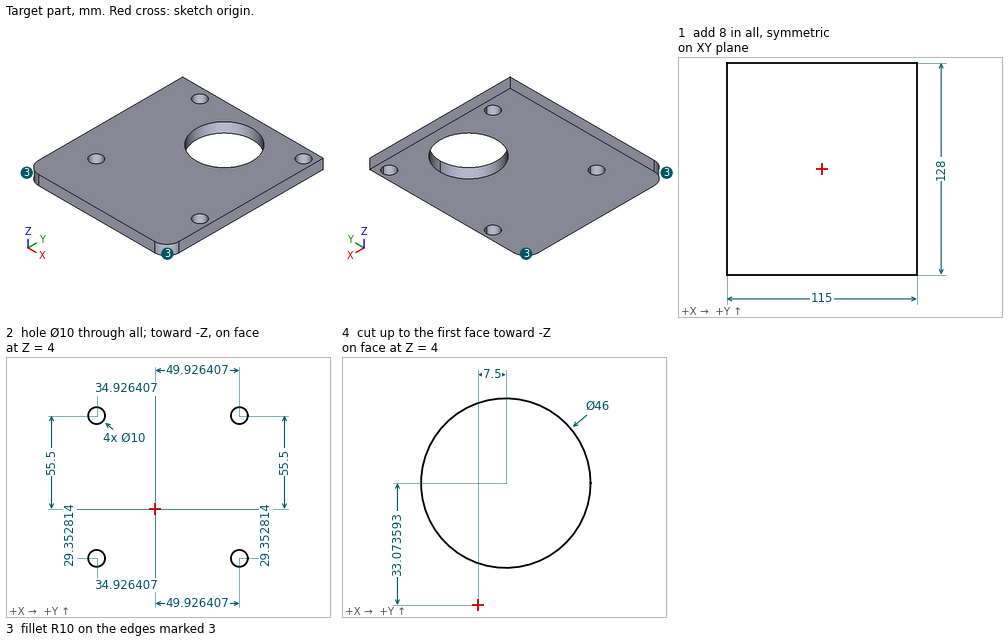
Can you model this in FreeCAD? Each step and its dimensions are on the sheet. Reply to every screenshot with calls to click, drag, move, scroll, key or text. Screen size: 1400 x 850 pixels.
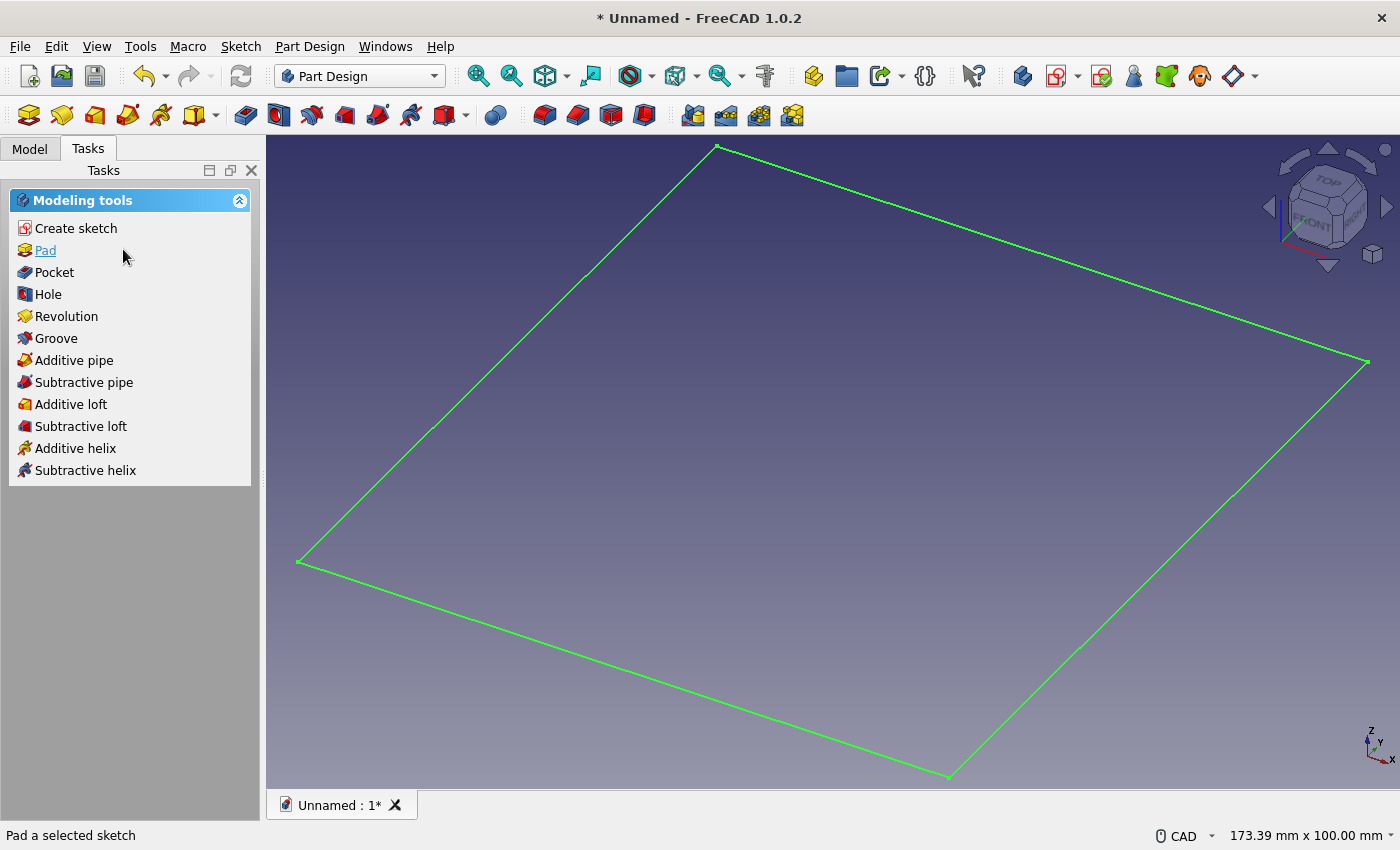
click(29, 116)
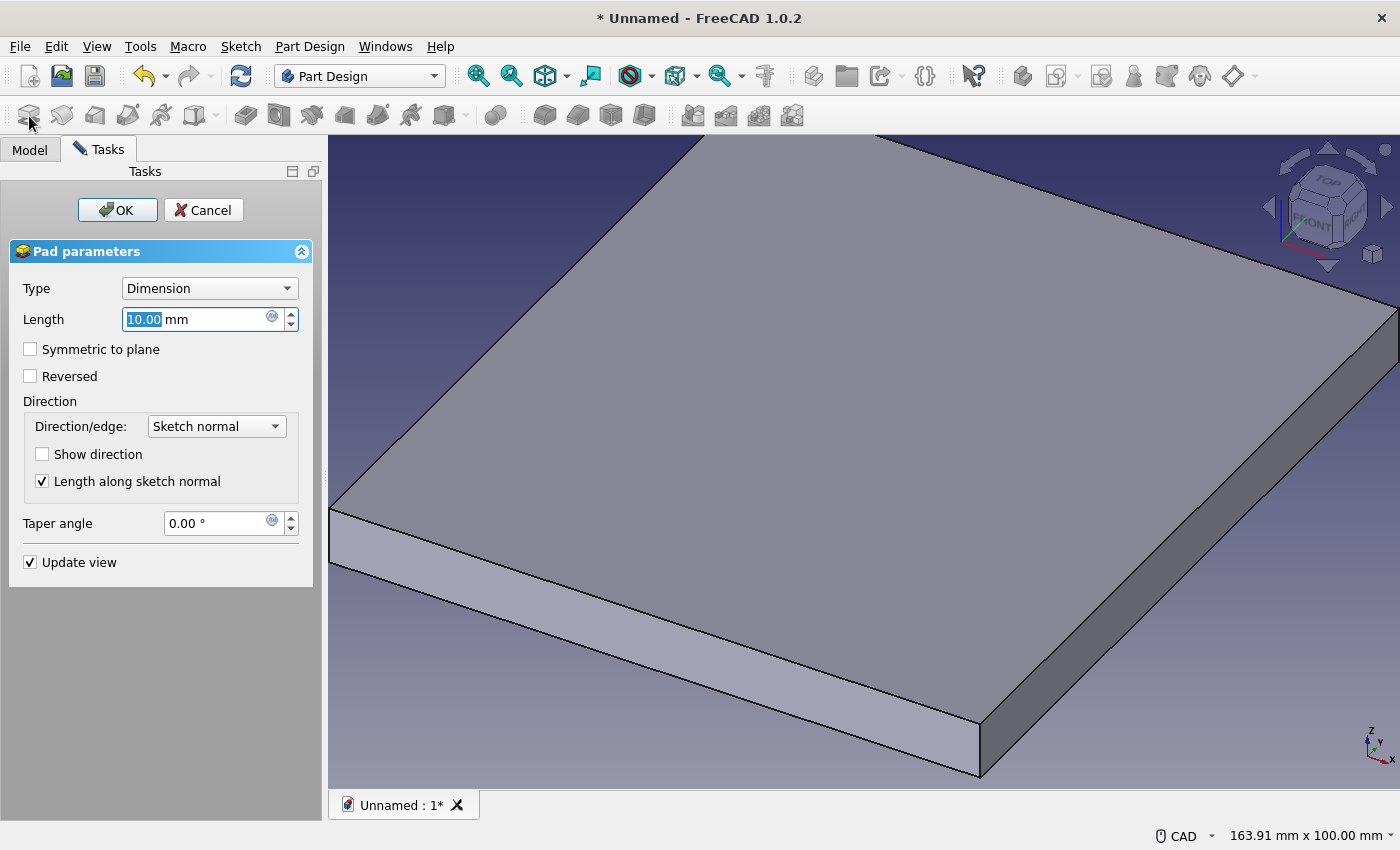
text(8)
key(Tab)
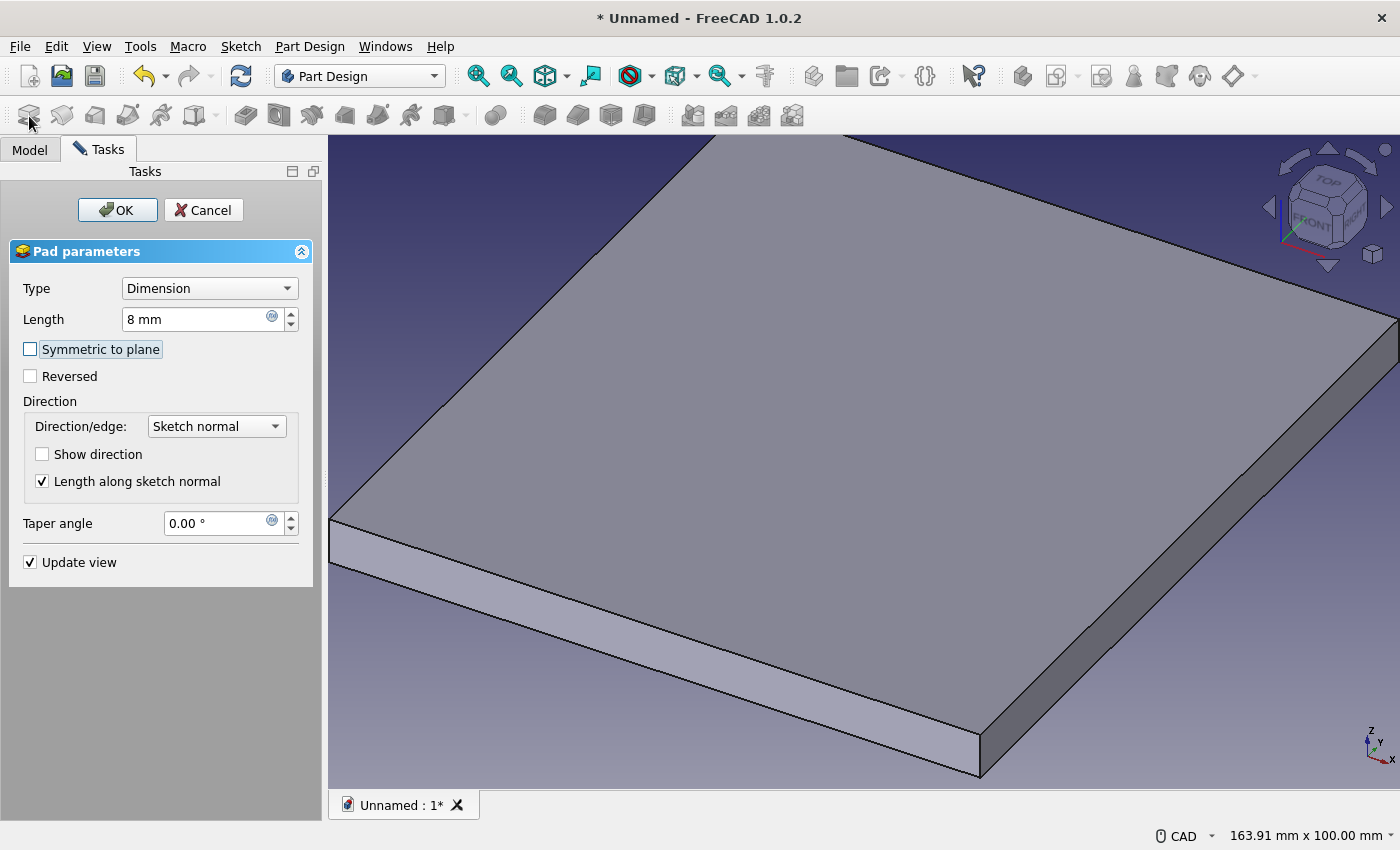
click(31, 349)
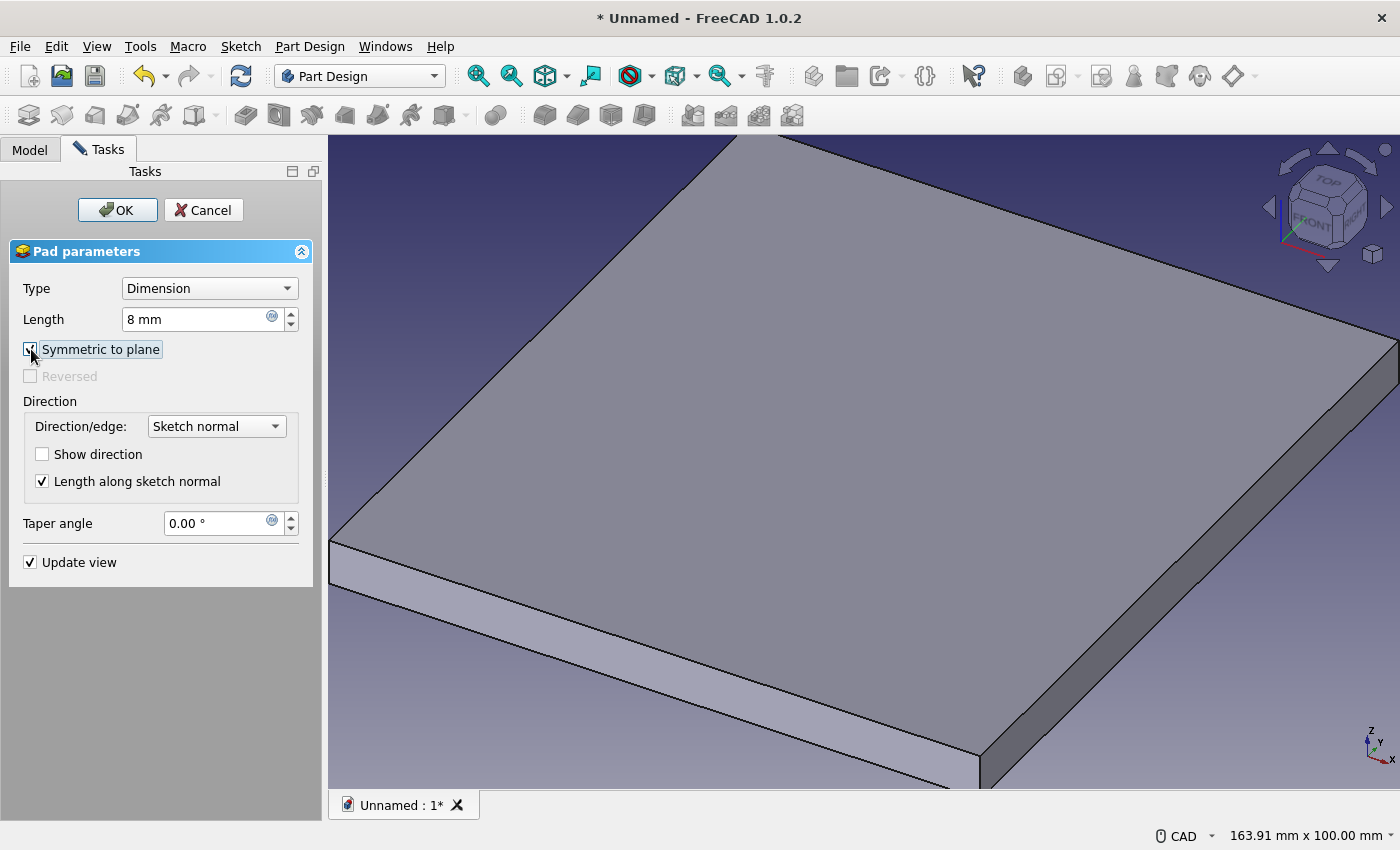
click(118, 210)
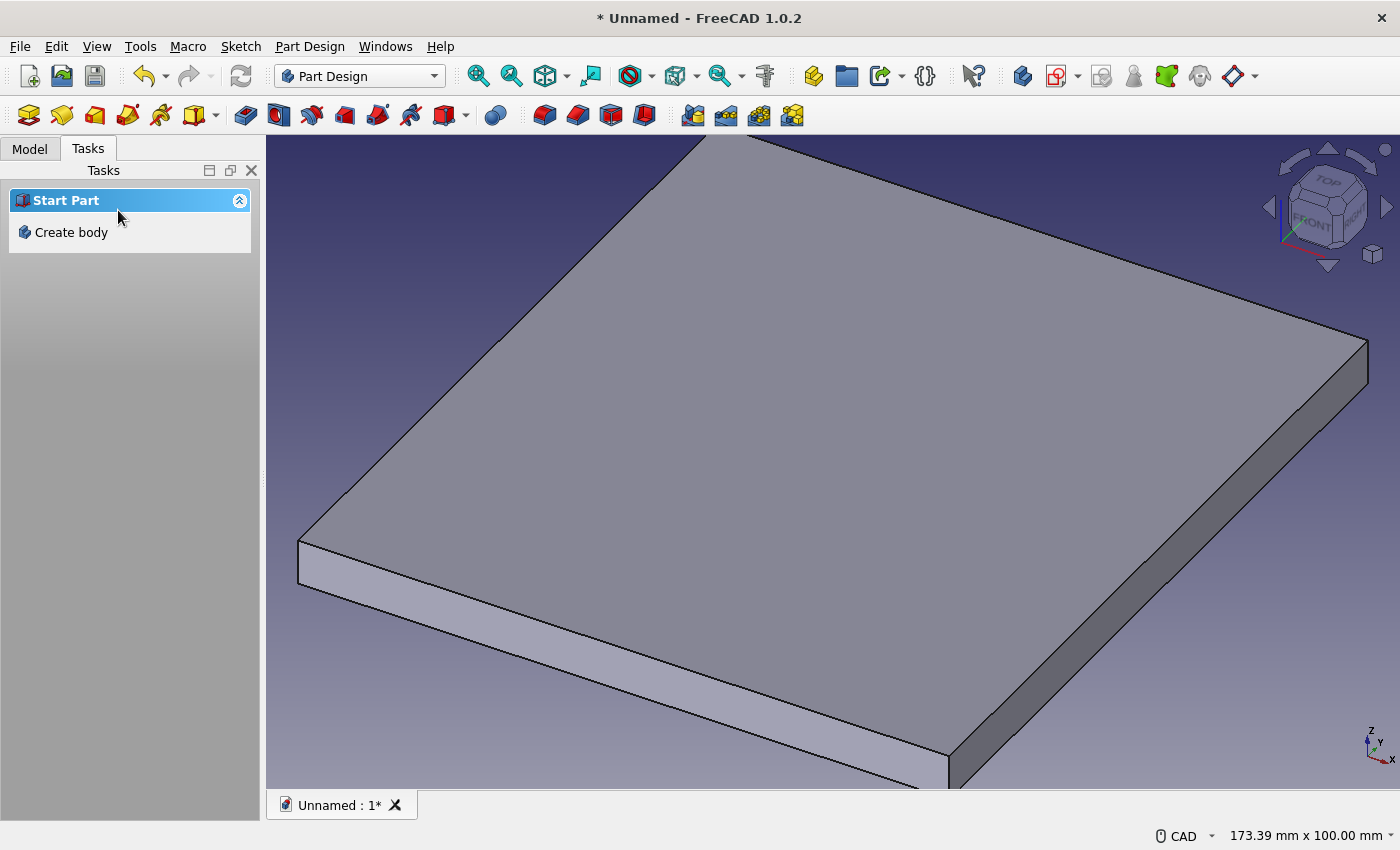
click(479, 76)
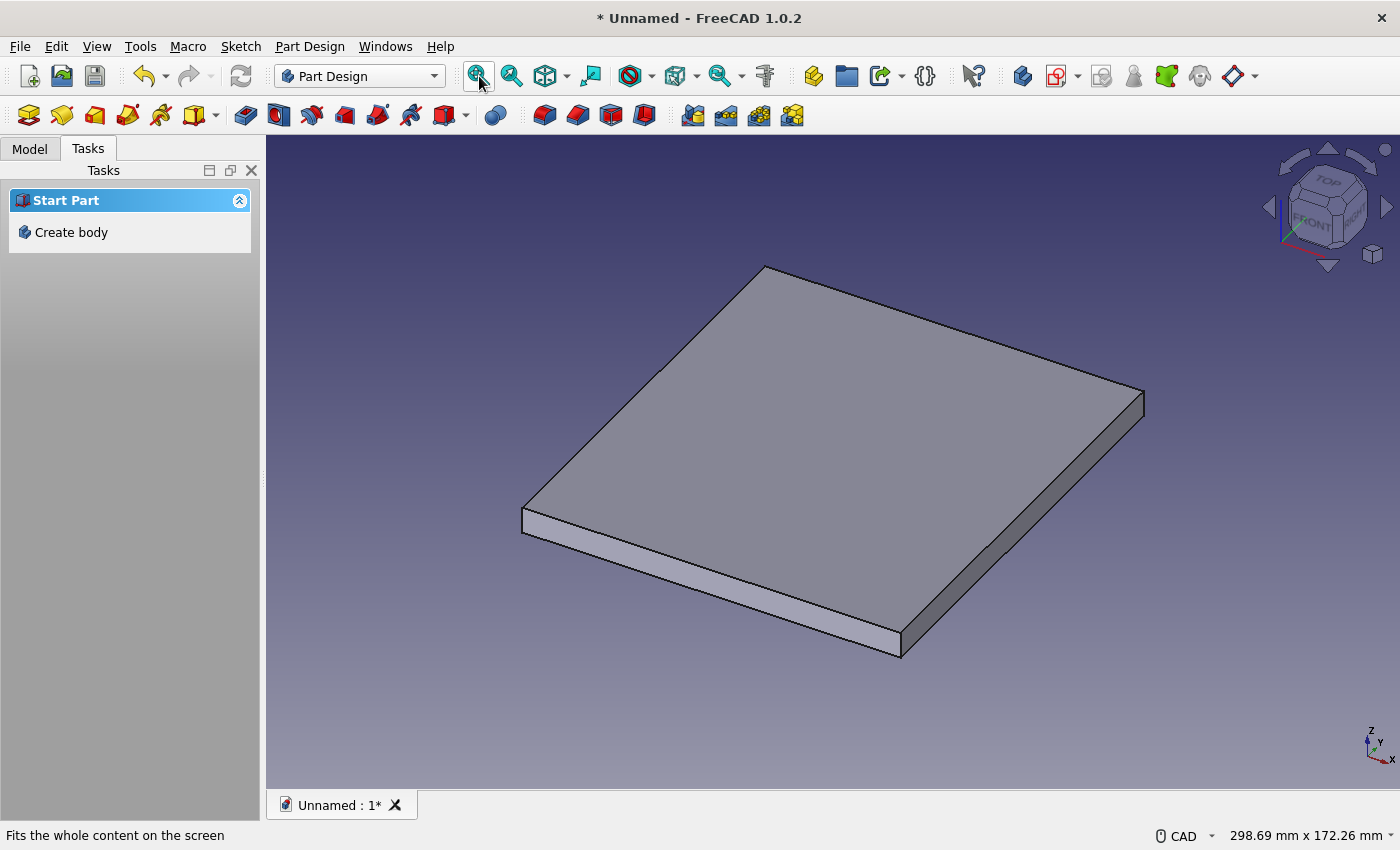
click(833, 449)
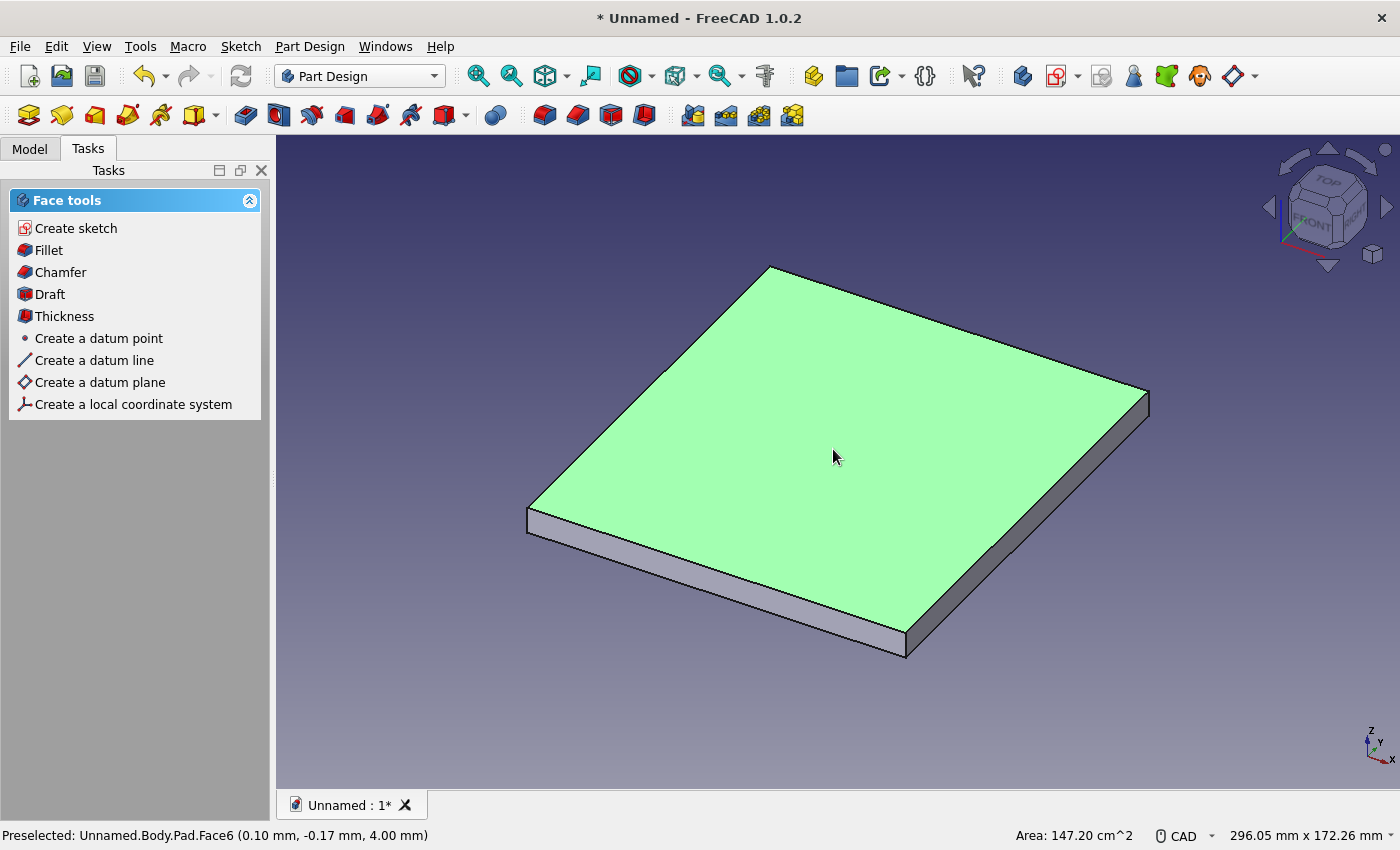
click(1056, 76)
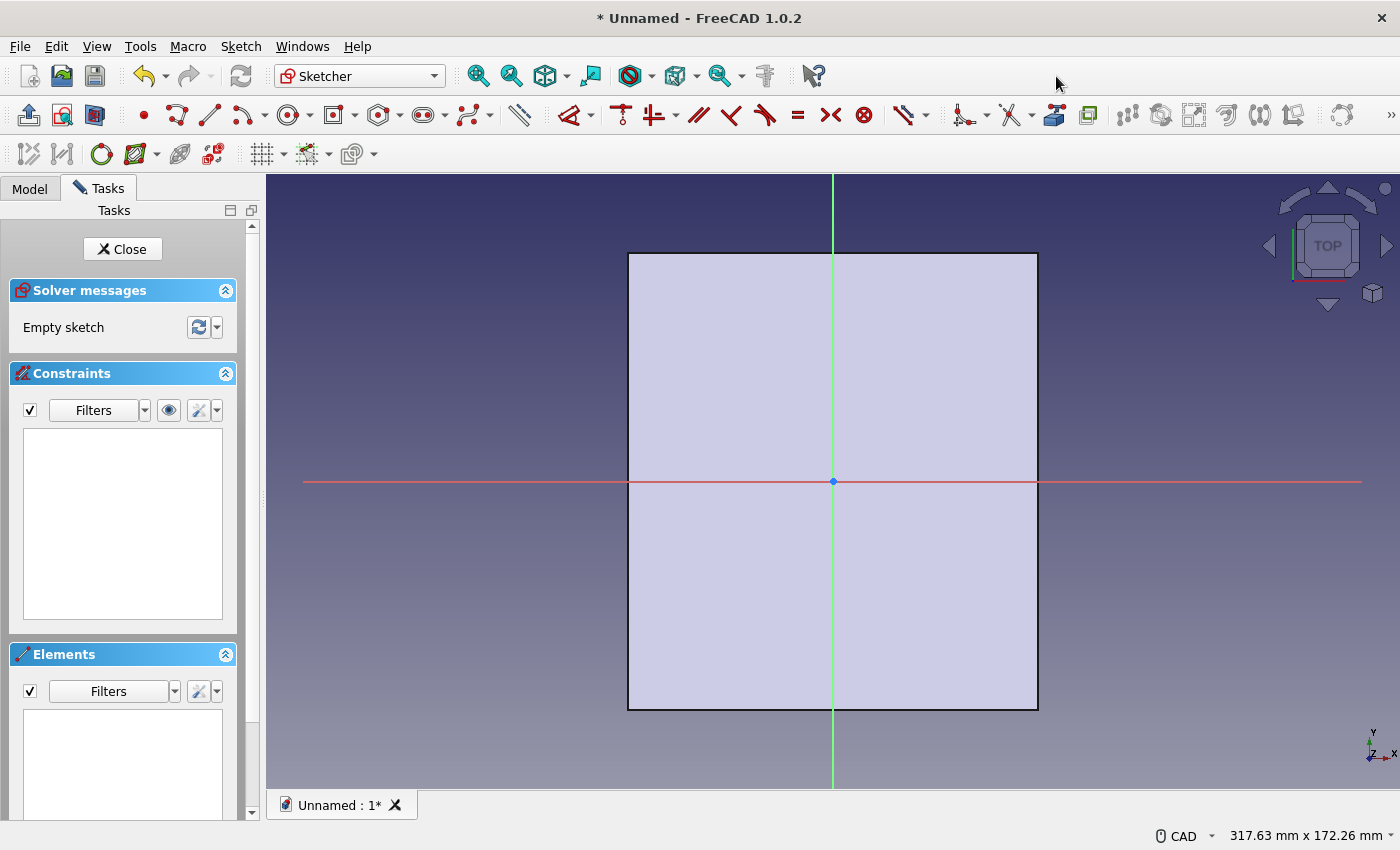
click(288, 116)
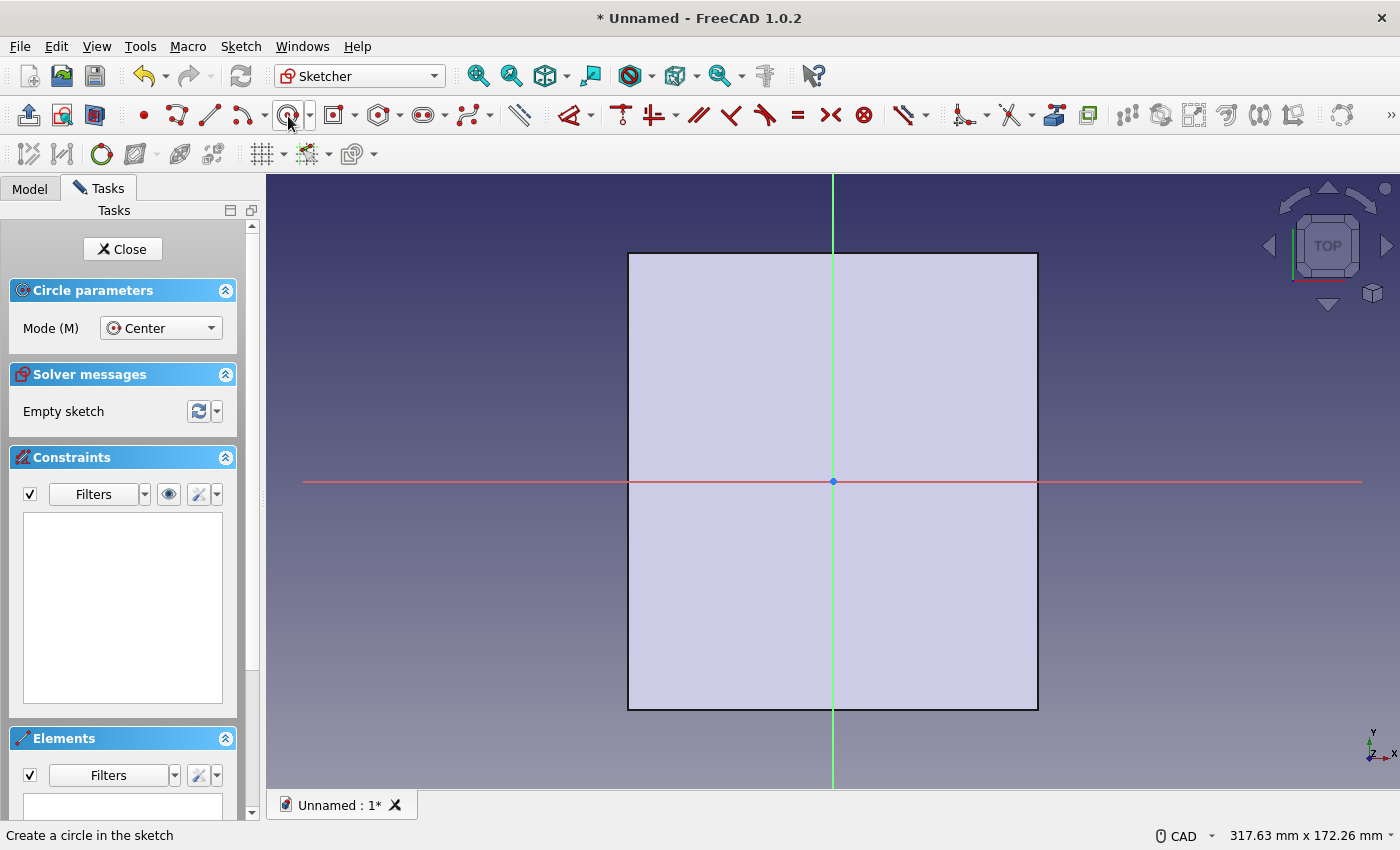
scroll(708, 283, up, 2)